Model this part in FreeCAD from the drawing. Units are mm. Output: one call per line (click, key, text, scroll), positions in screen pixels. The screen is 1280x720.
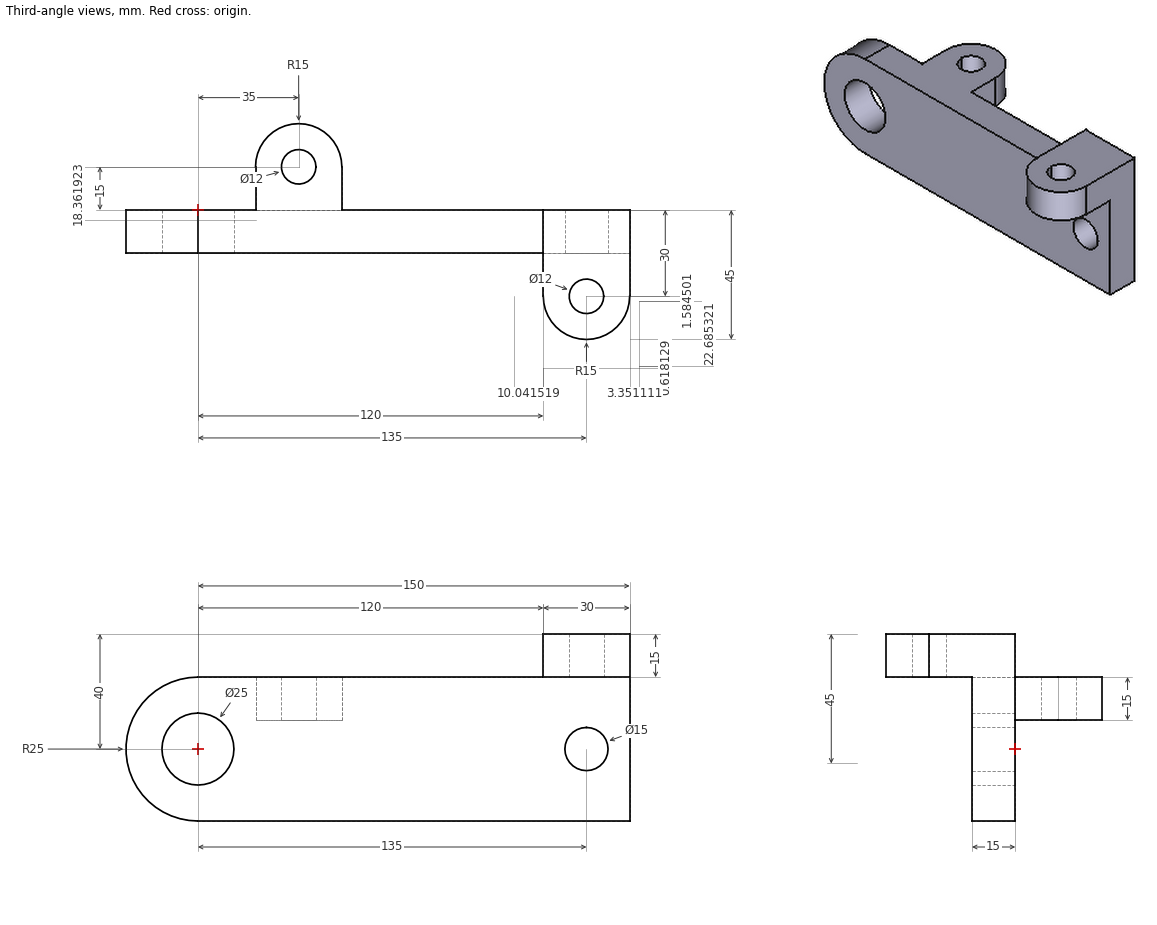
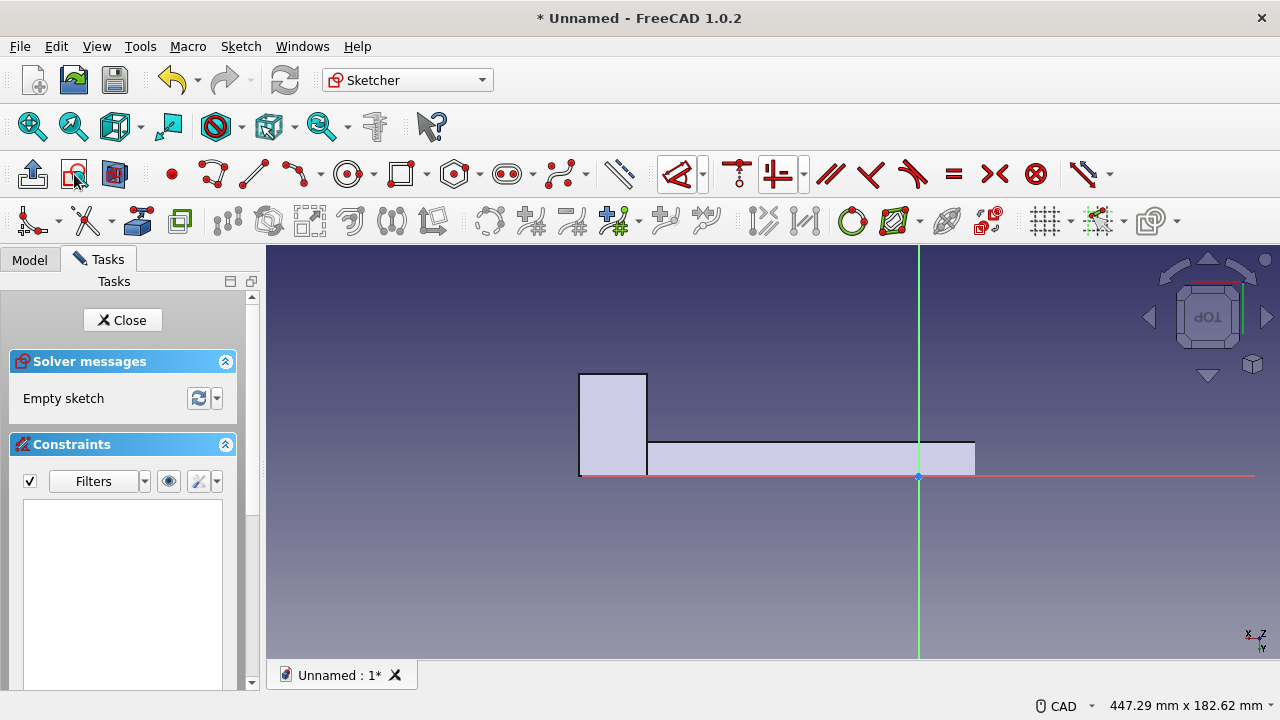
scroll(584, 358, up, 6)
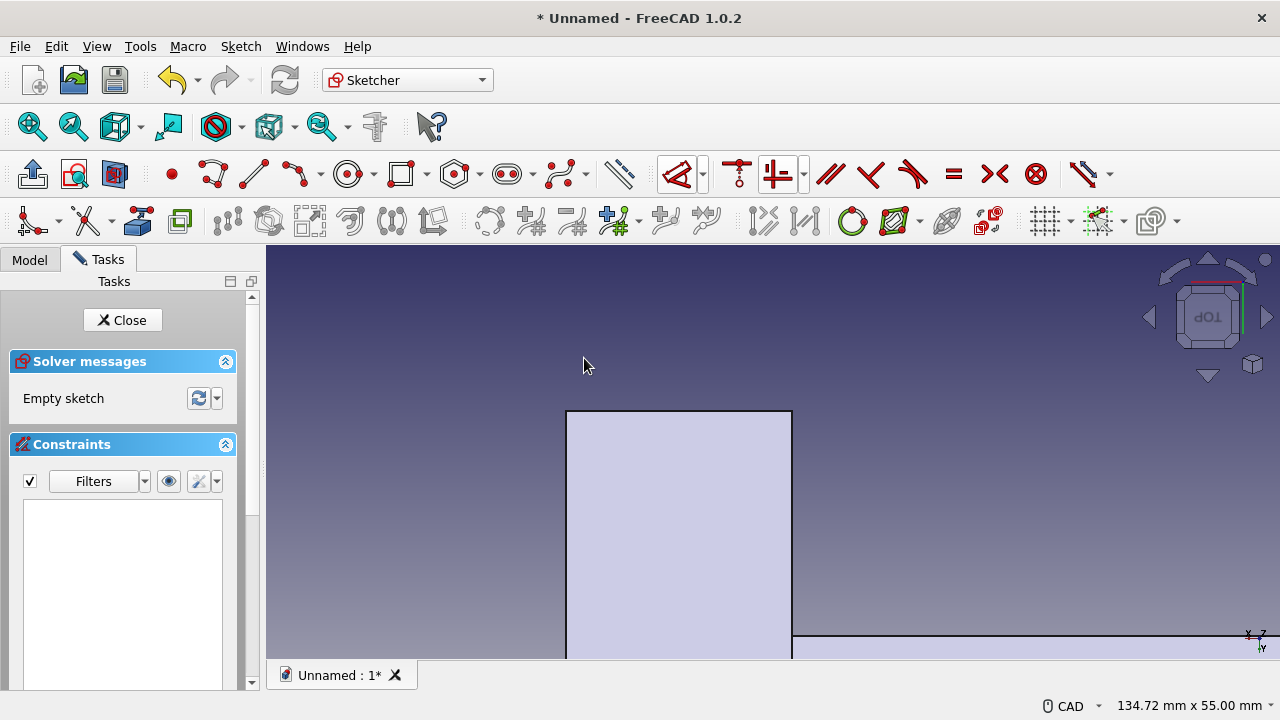
click(213, 174)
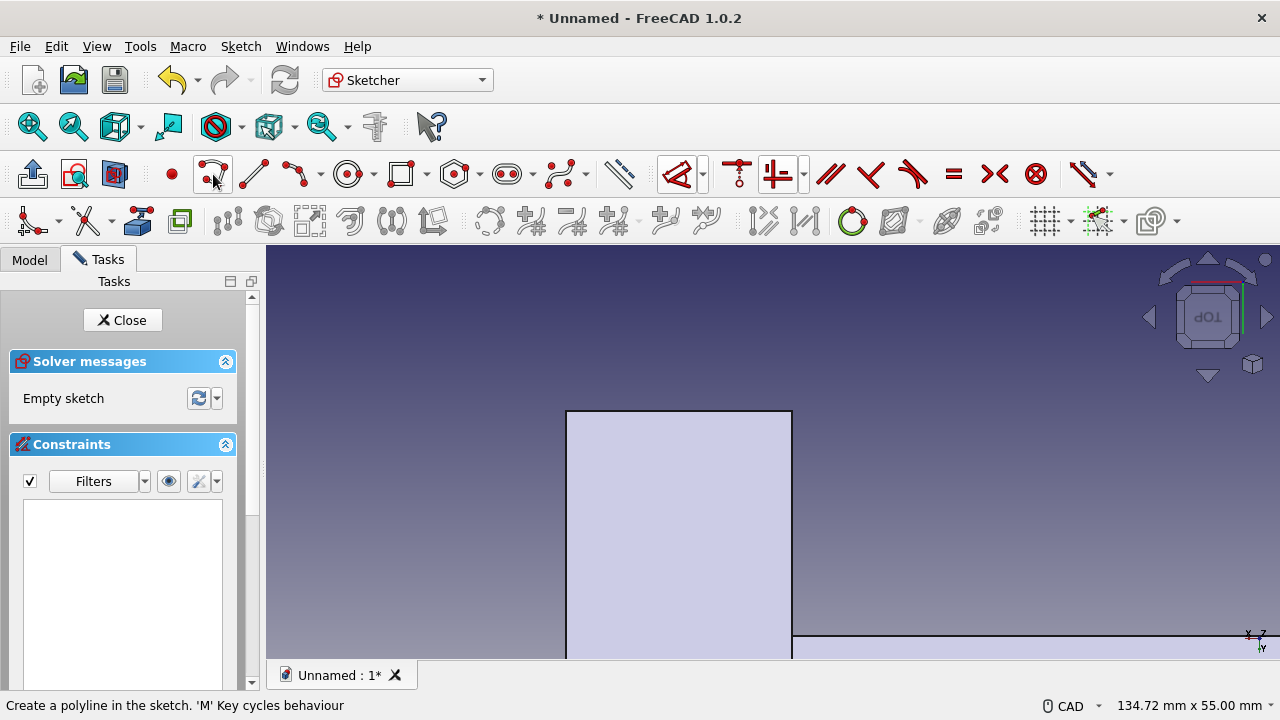
click(792, 524)
click(867, 524)
click(792, 336)
click(540, 349)
click(540, 512)
click(566, 524)
right_click(566, 524)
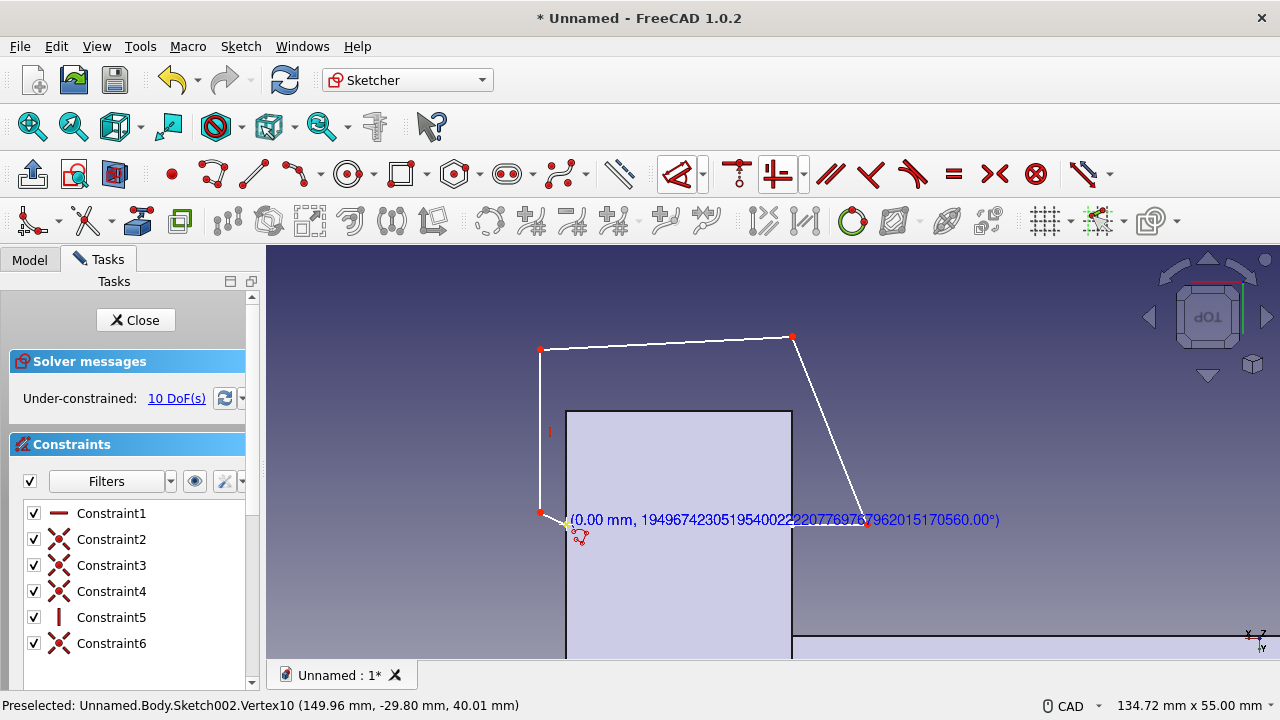
click(294, 174)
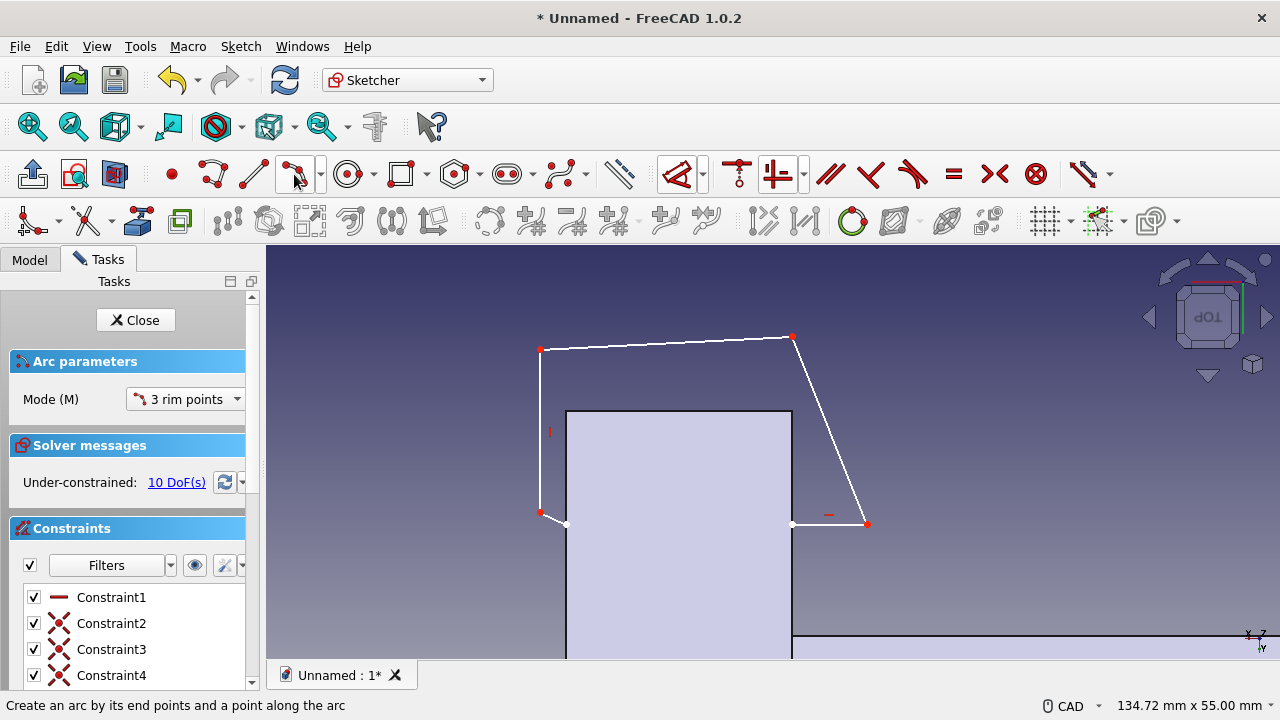
click(566, 525)
click(792, 525)
click(679, 411)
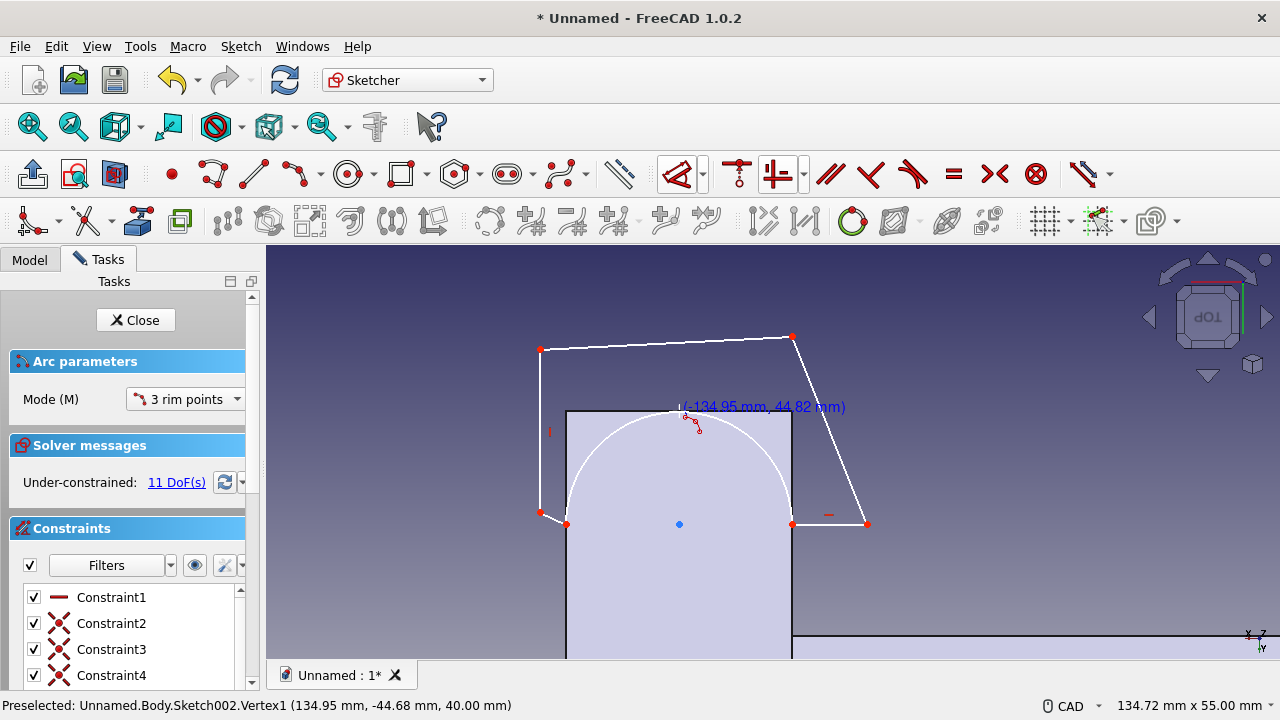
click(348, 174)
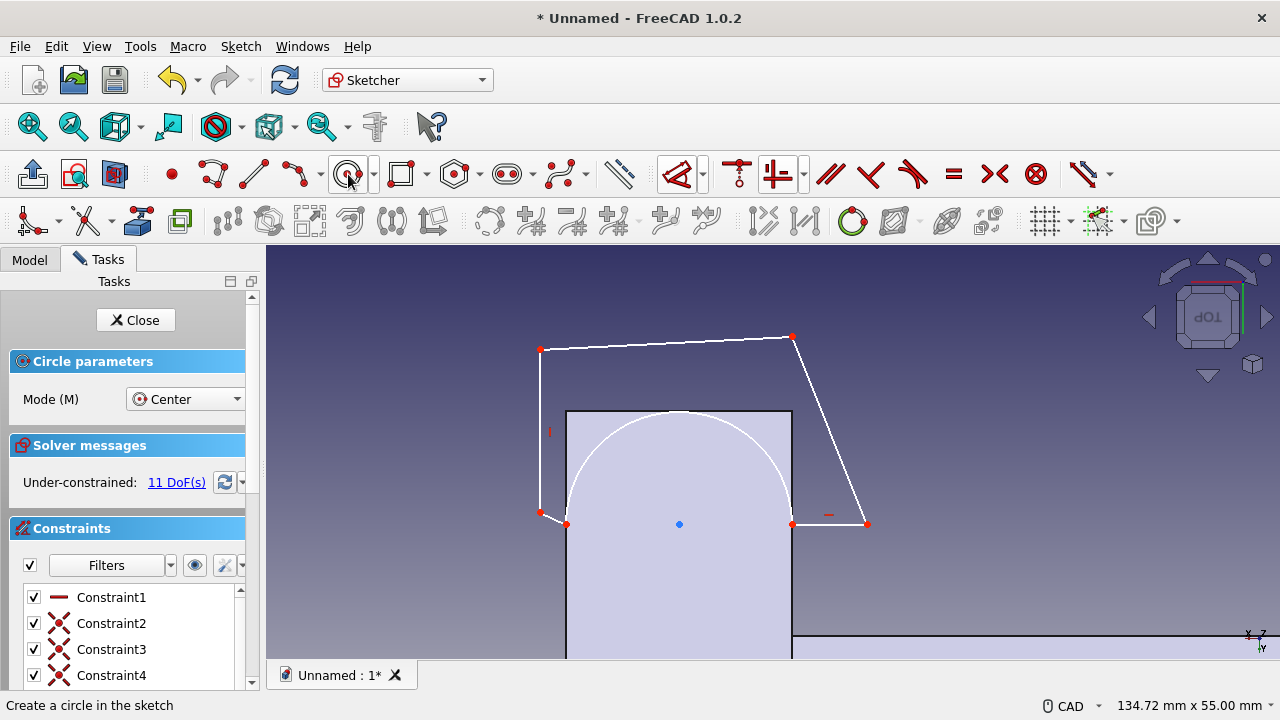
click(679, 524)
click(711, 492)
key(Escape)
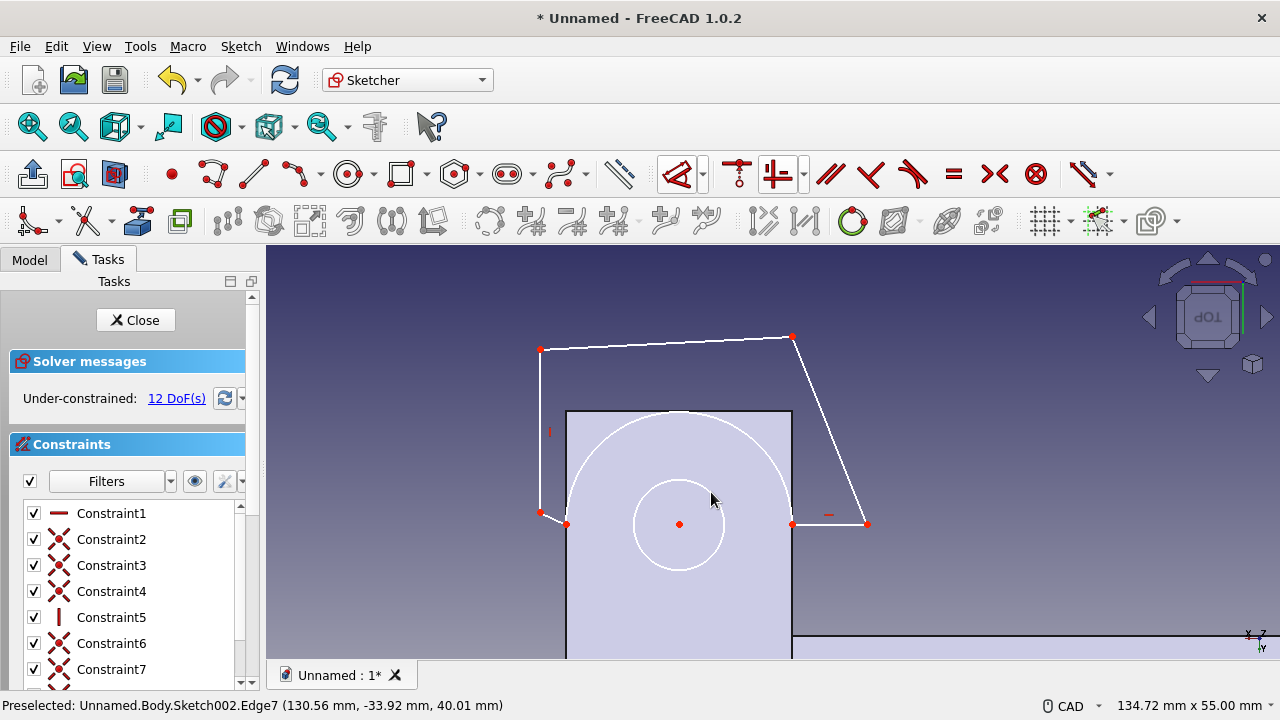
click(745, 434)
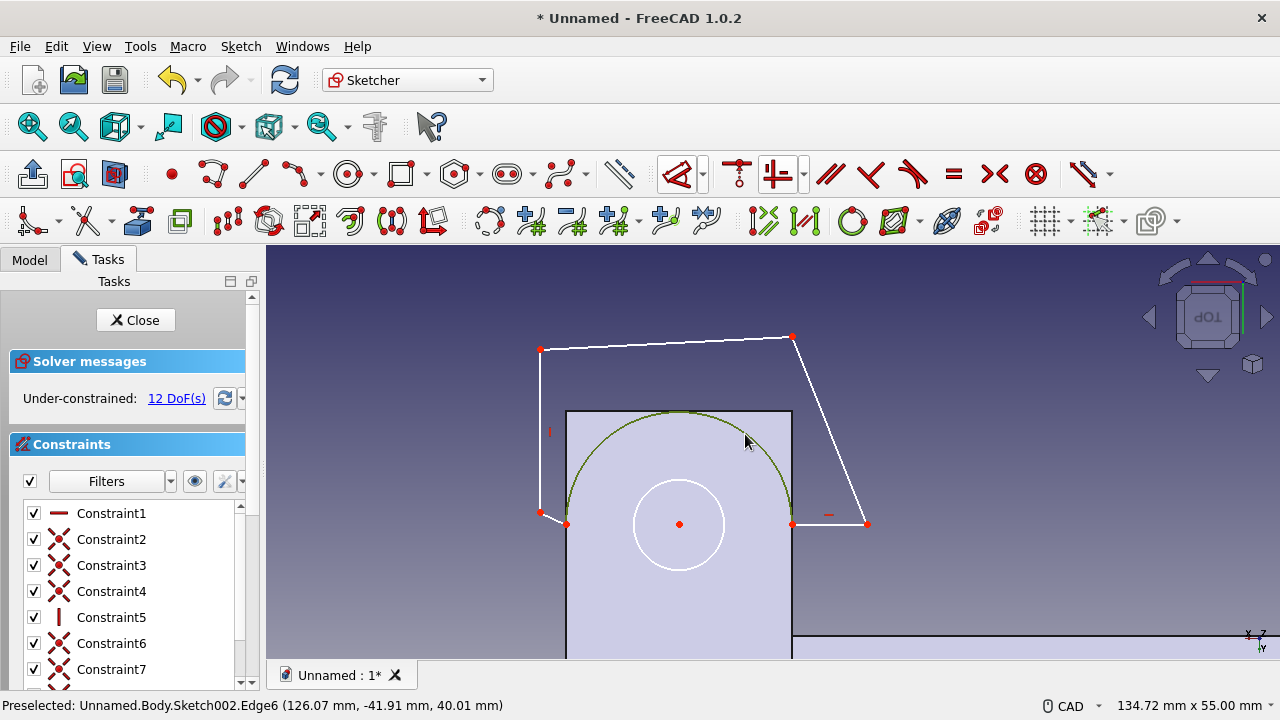
click(702, 174)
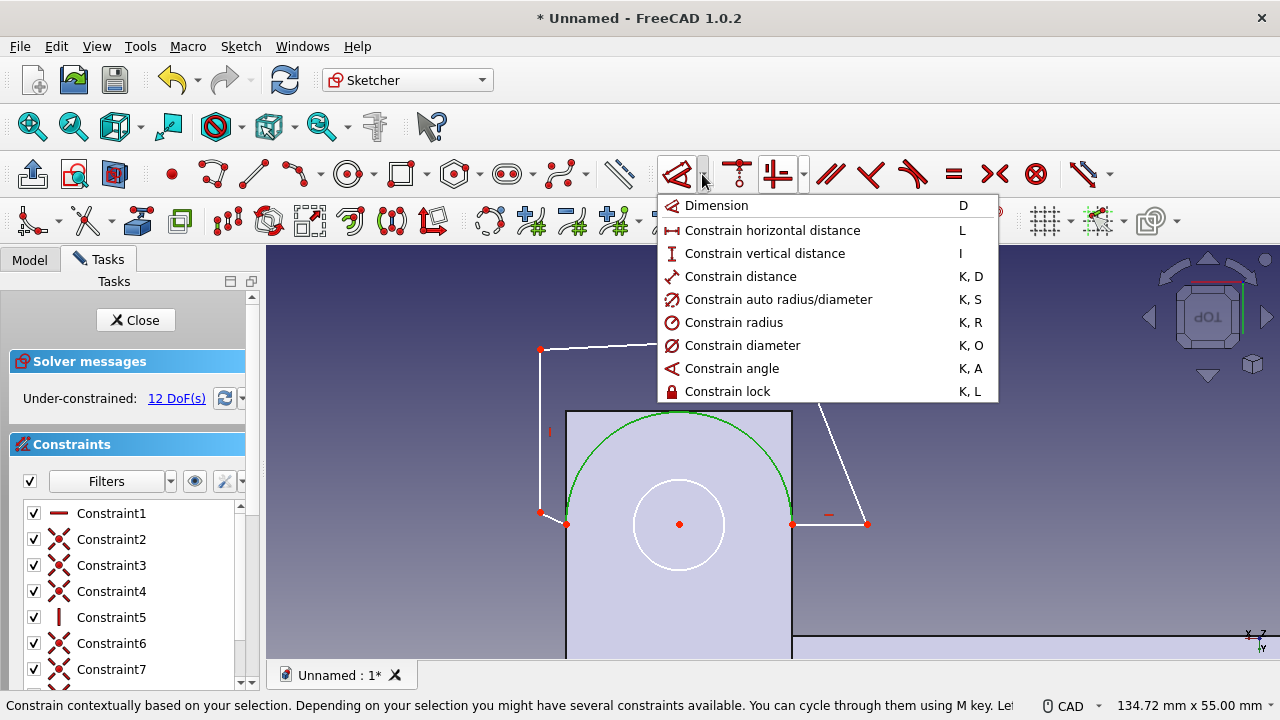
click(828, 322)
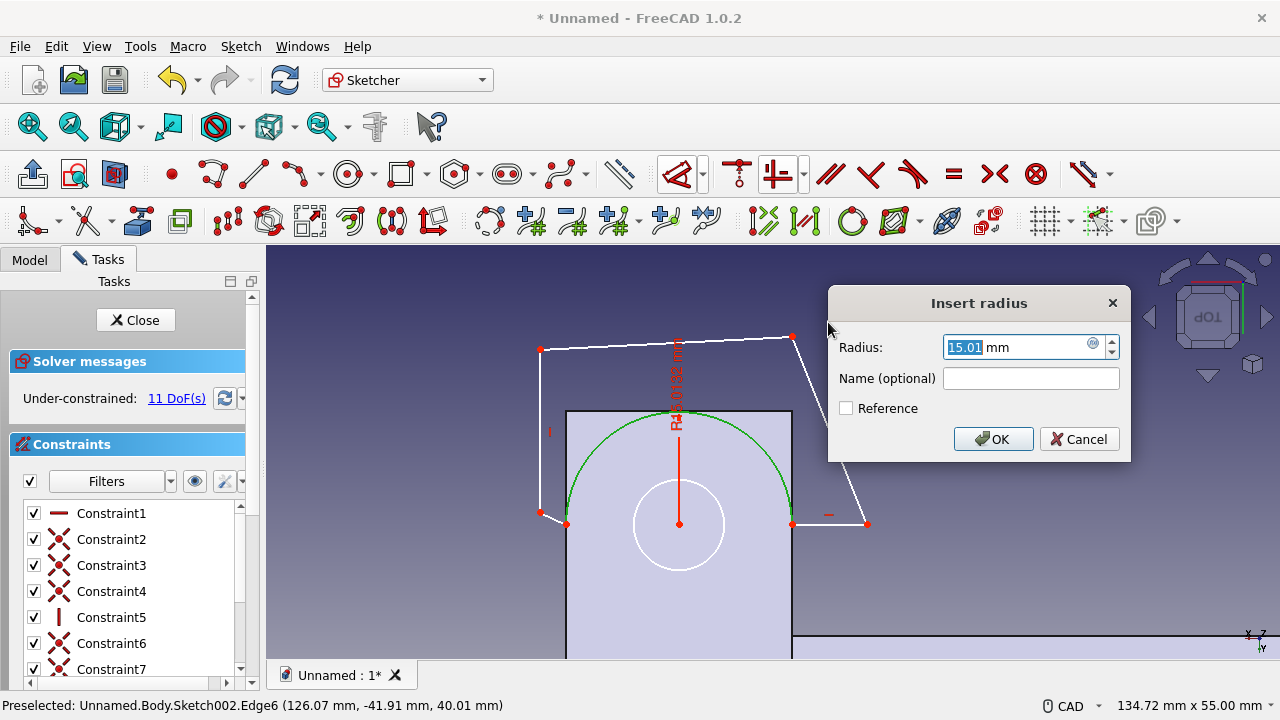
text(15)
key(Return)